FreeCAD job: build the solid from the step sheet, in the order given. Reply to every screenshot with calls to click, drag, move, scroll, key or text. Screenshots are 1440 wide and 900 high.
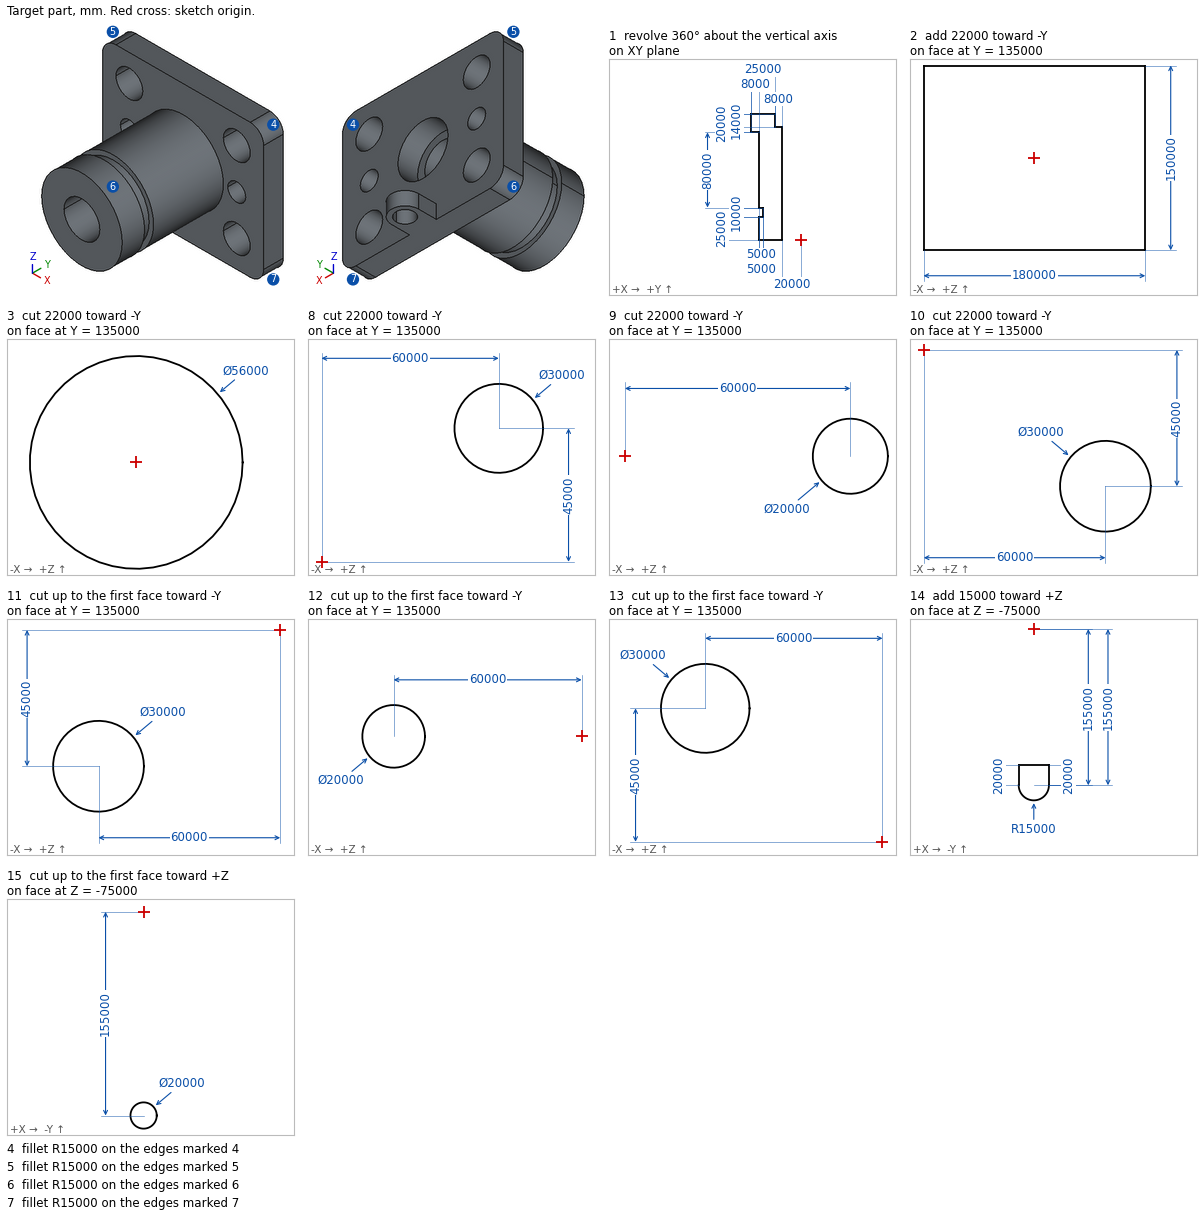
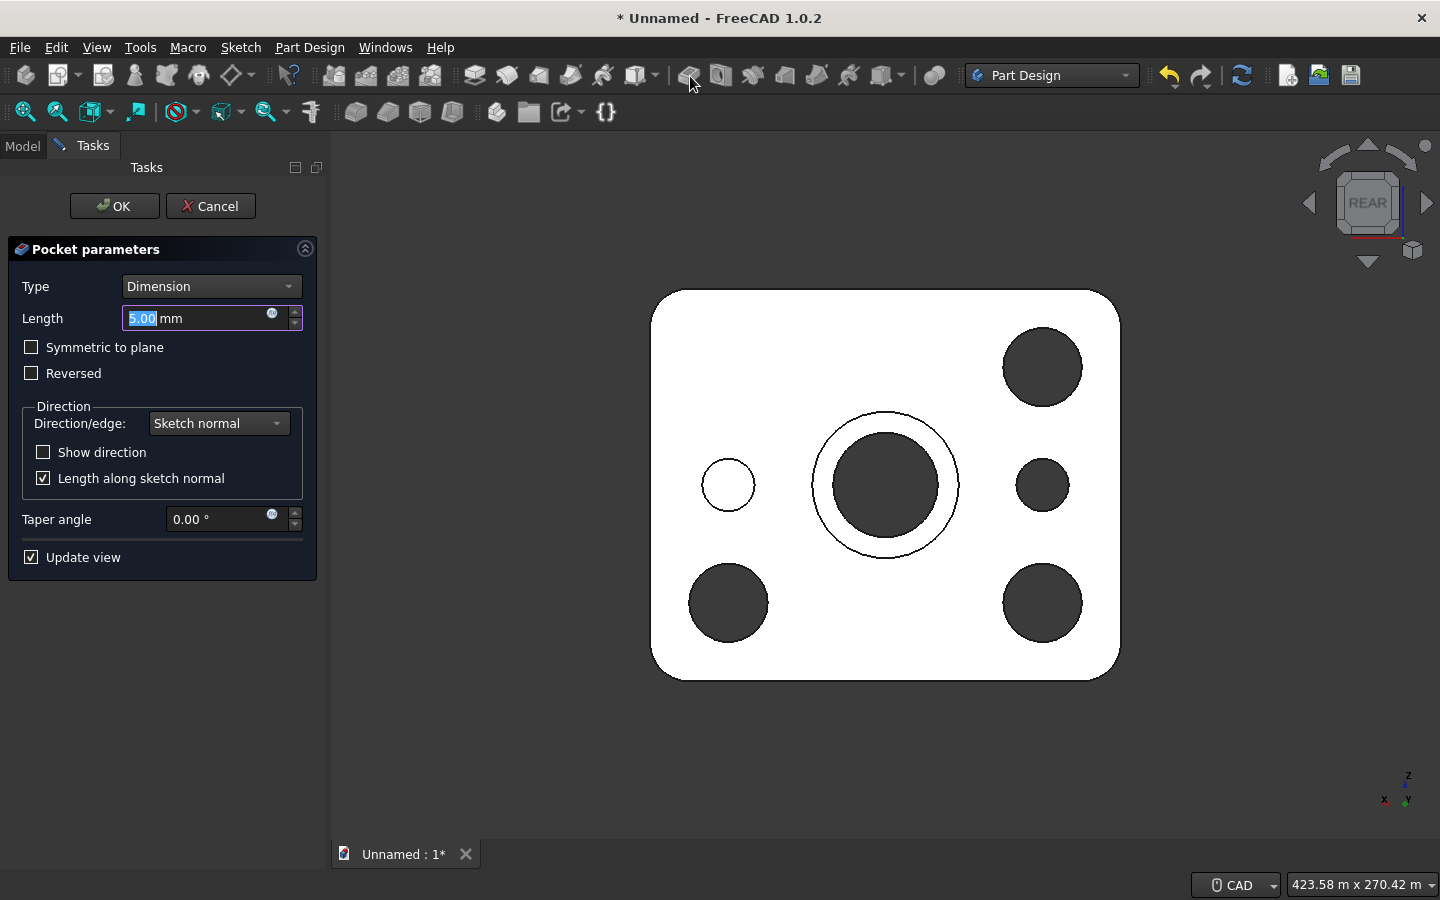
click(212, 286)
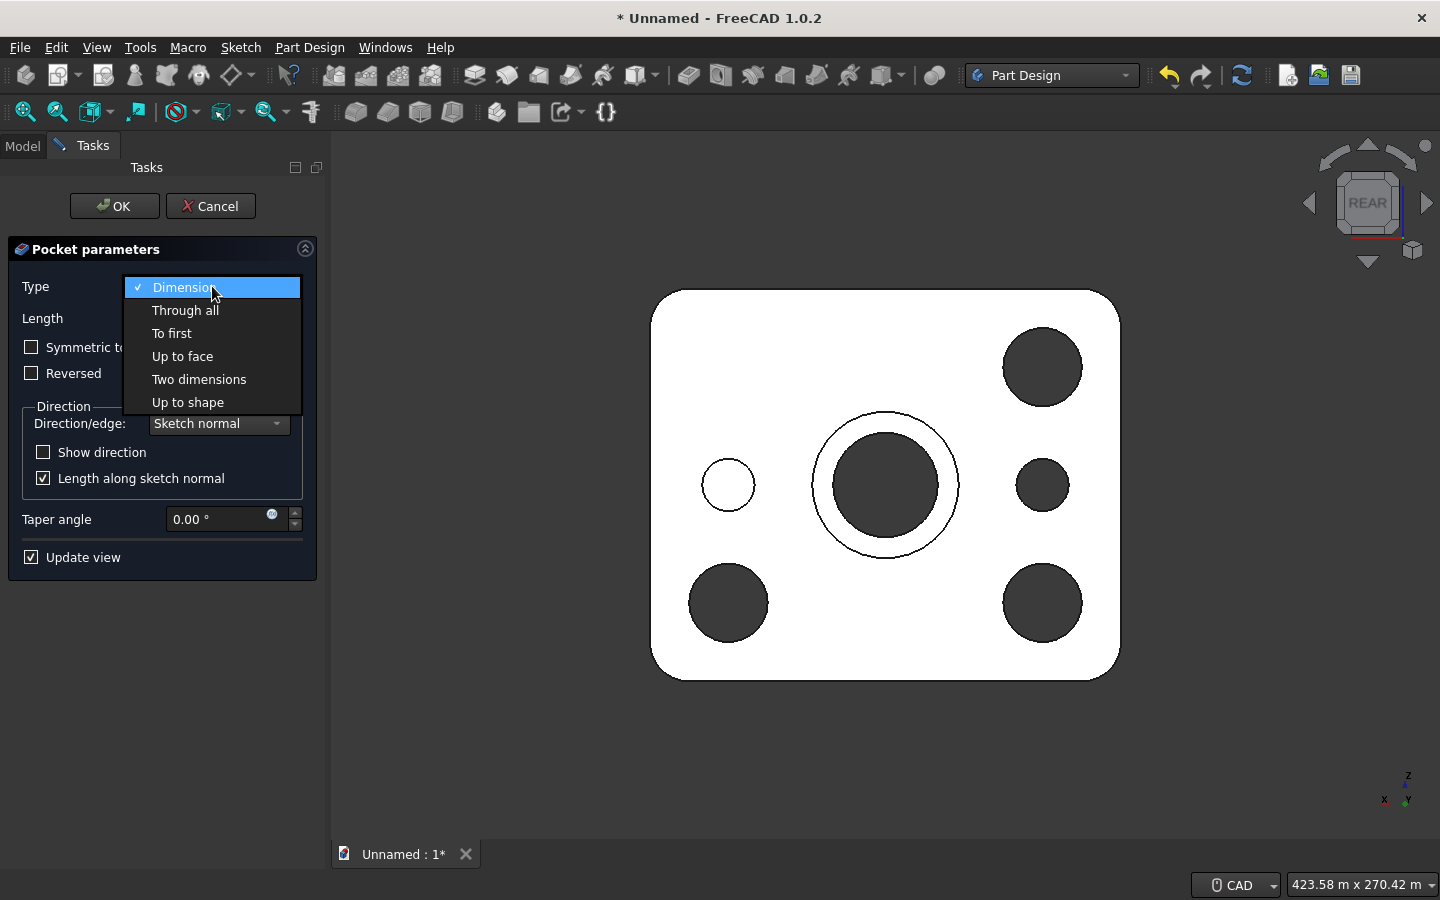
click(212, 334)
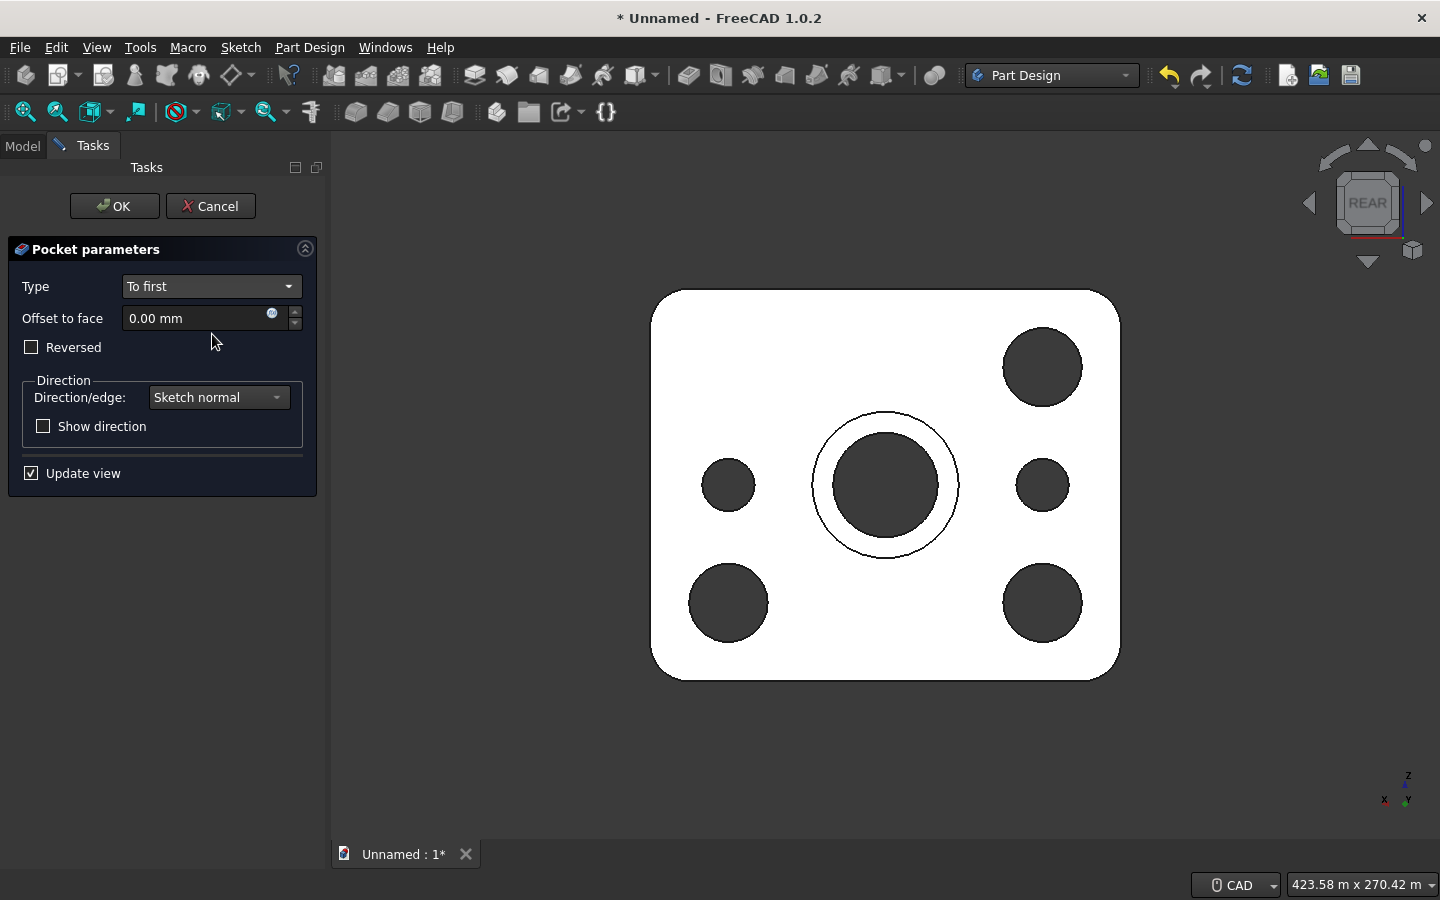
click(115, 206)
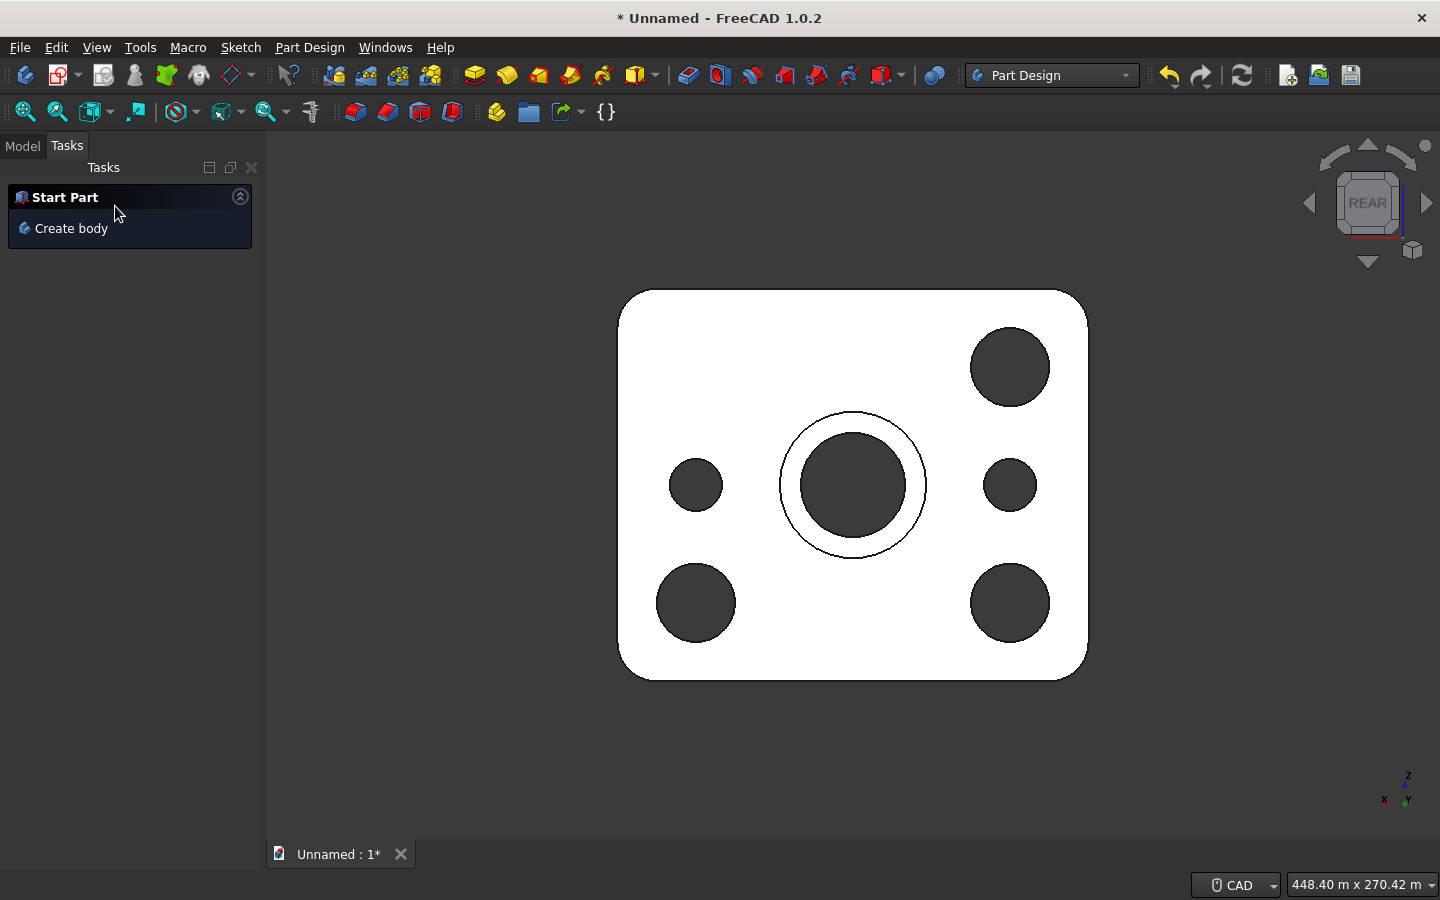
click(718, 372)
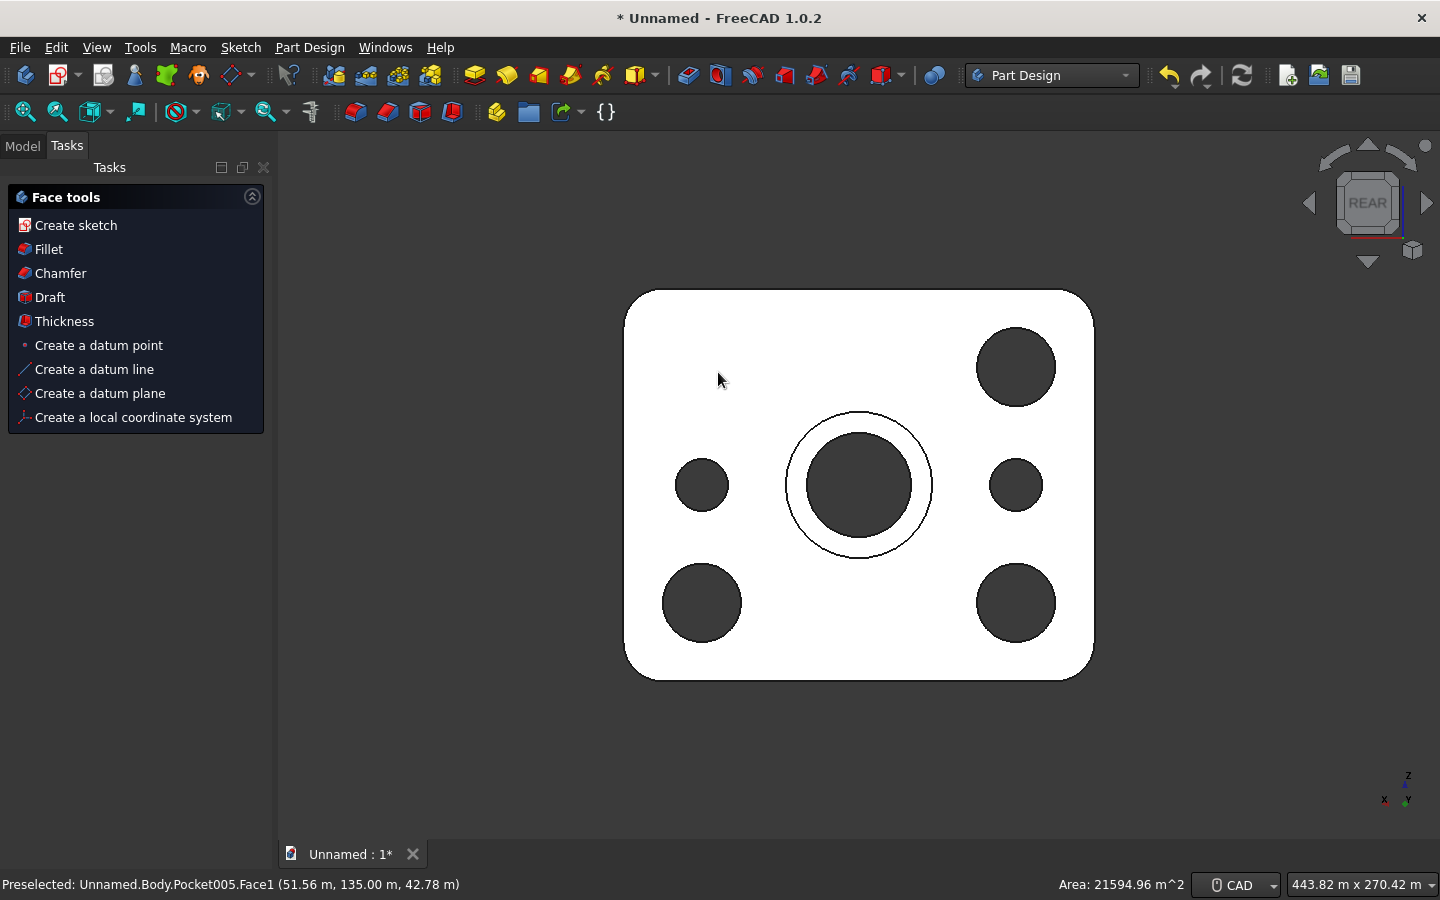
click(58, 76)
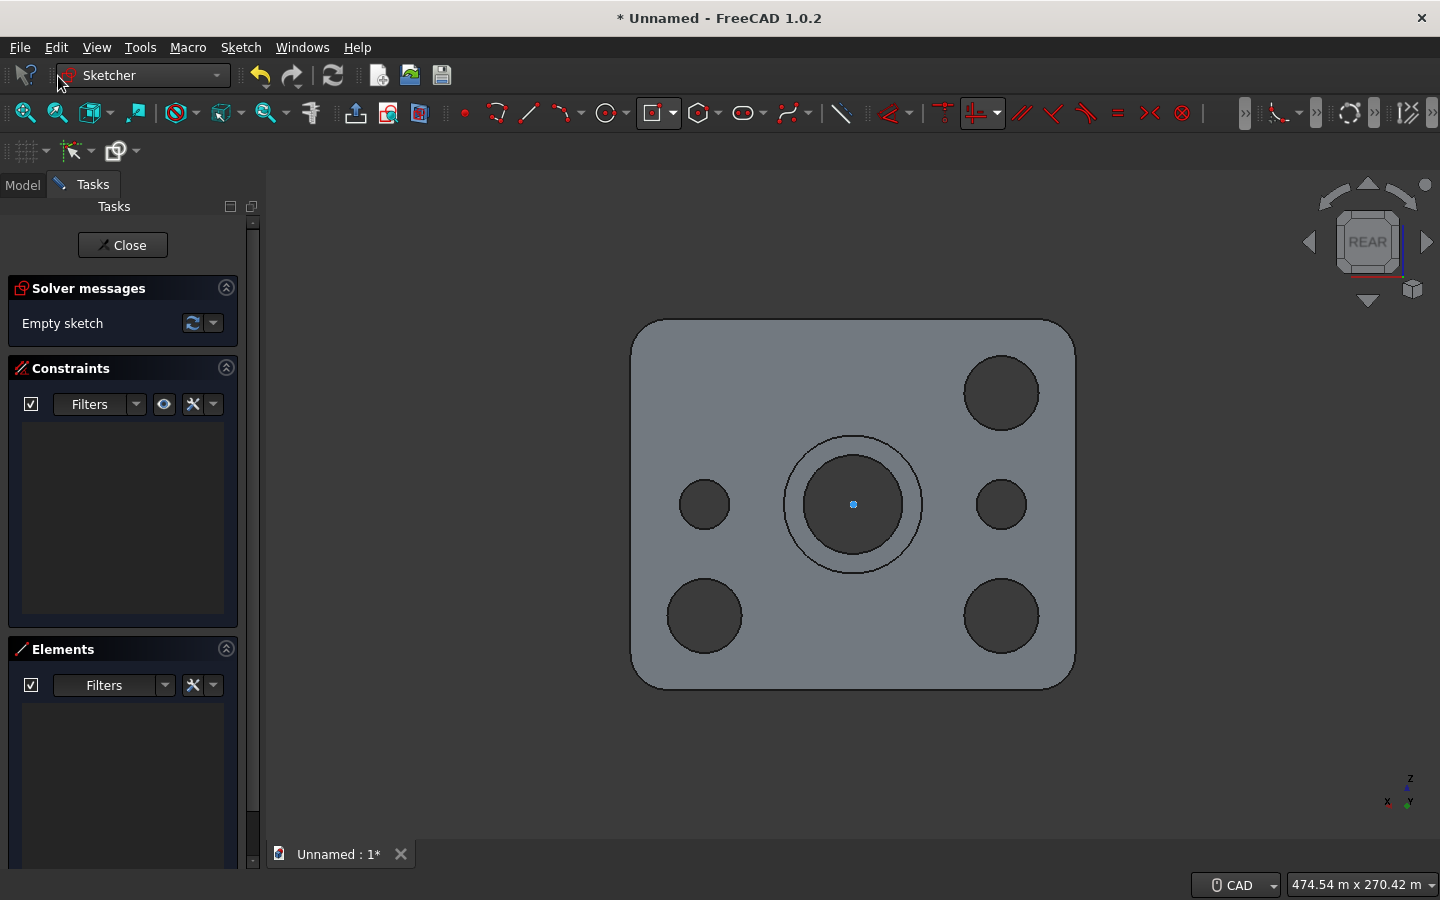
scroll(689, 371, up, 9)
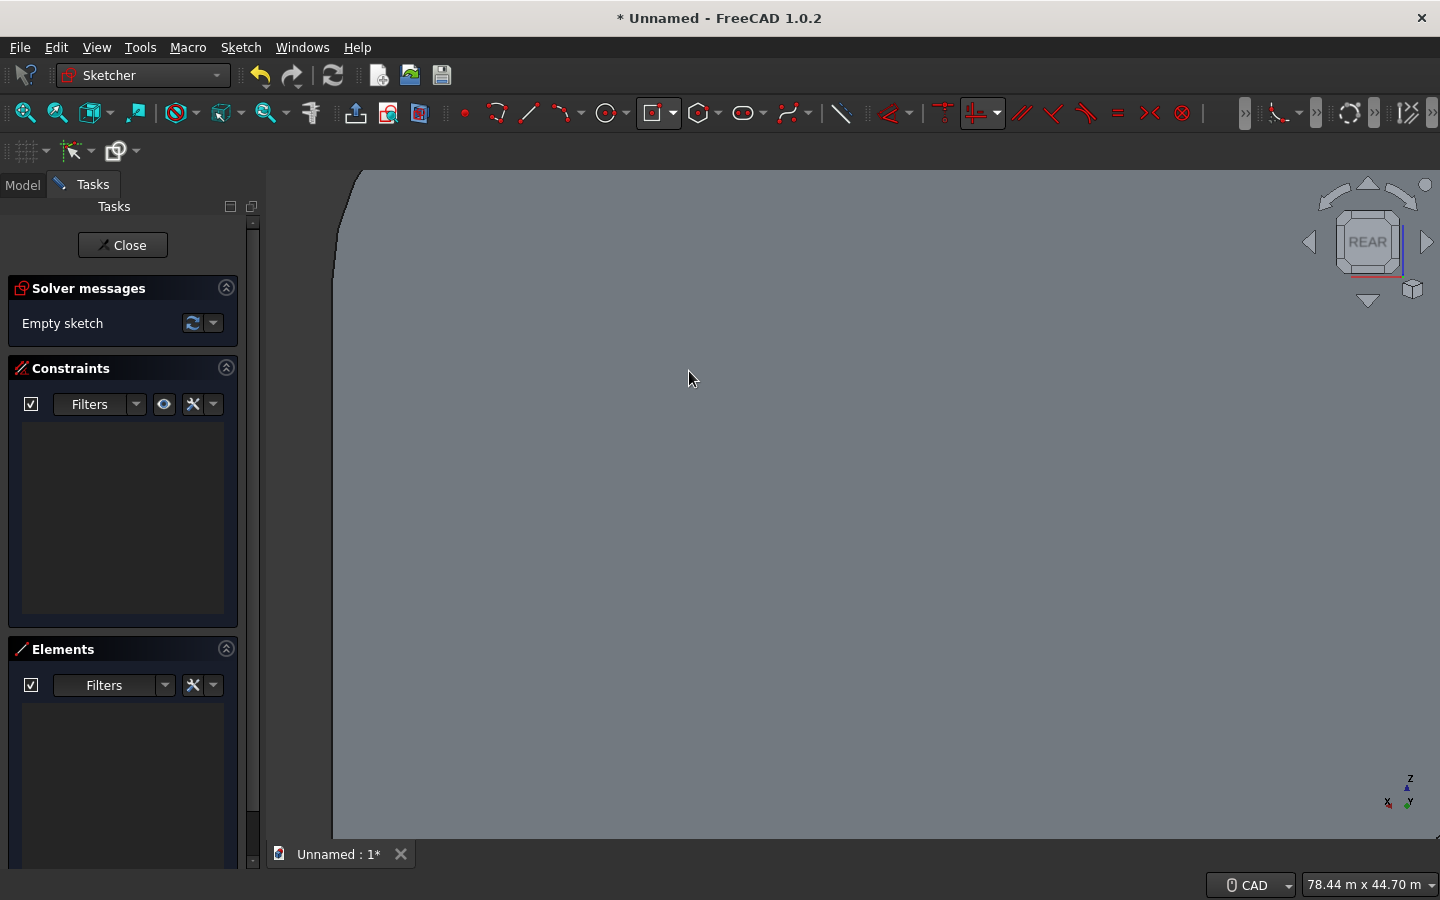
click(606, 114)